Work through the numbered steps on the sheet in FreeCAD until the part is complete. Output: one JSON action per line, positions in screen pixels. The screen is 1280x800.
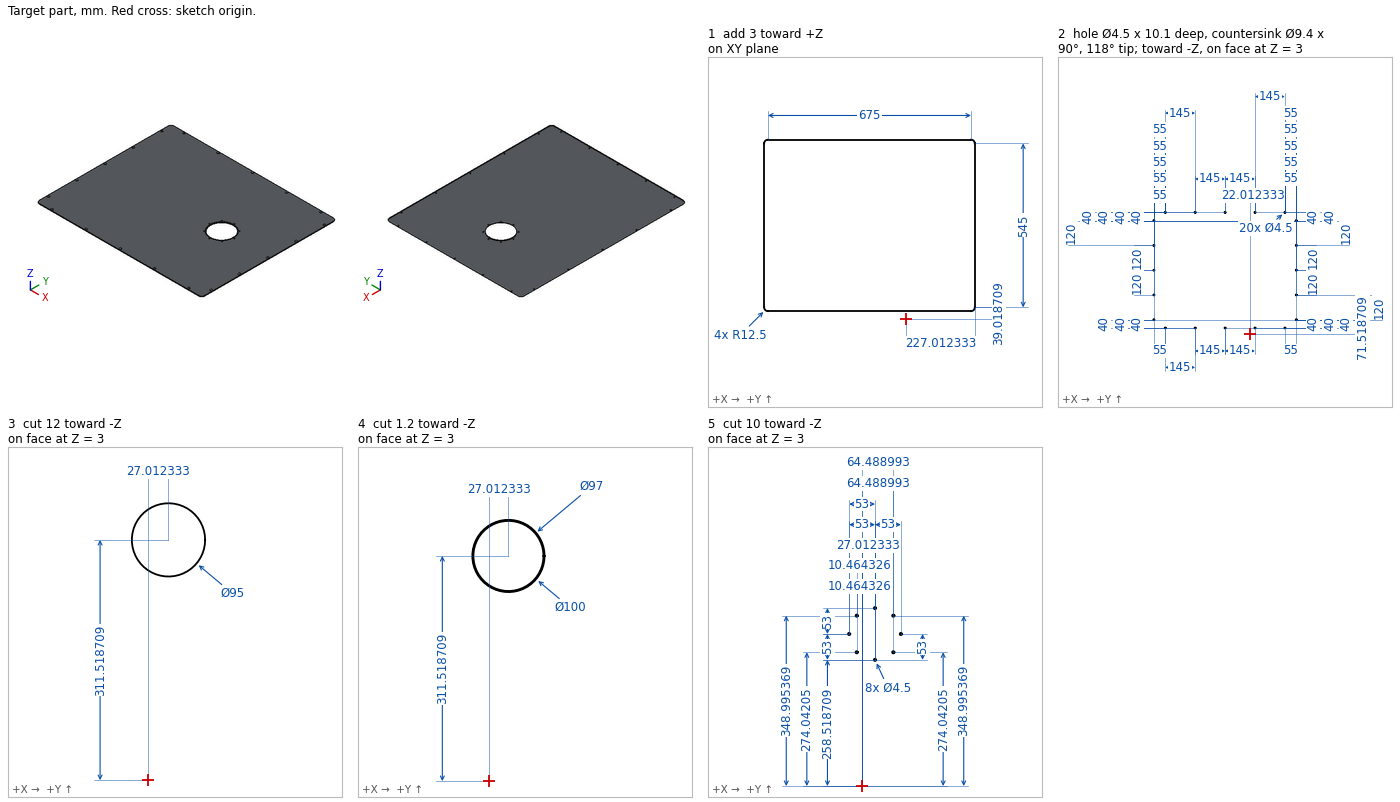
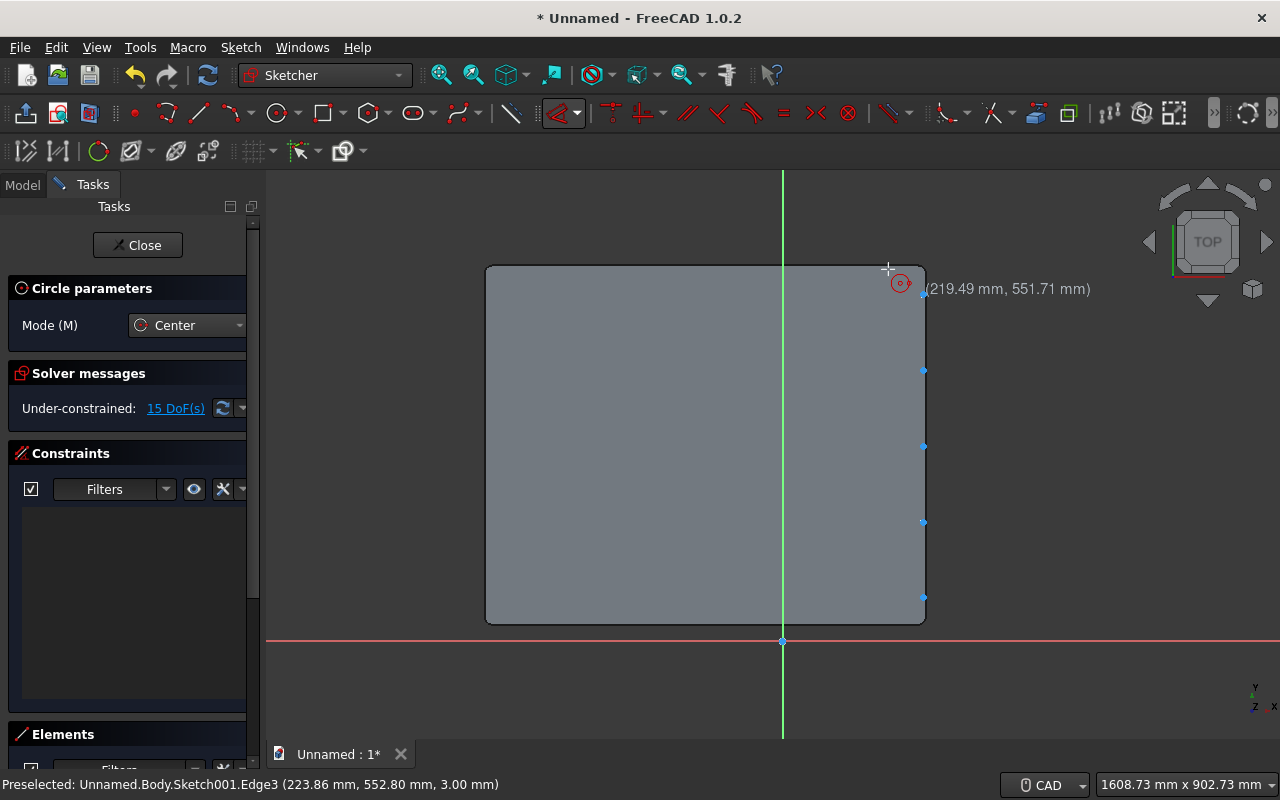
{"action": "left_click", "coordinate": [888, 269]}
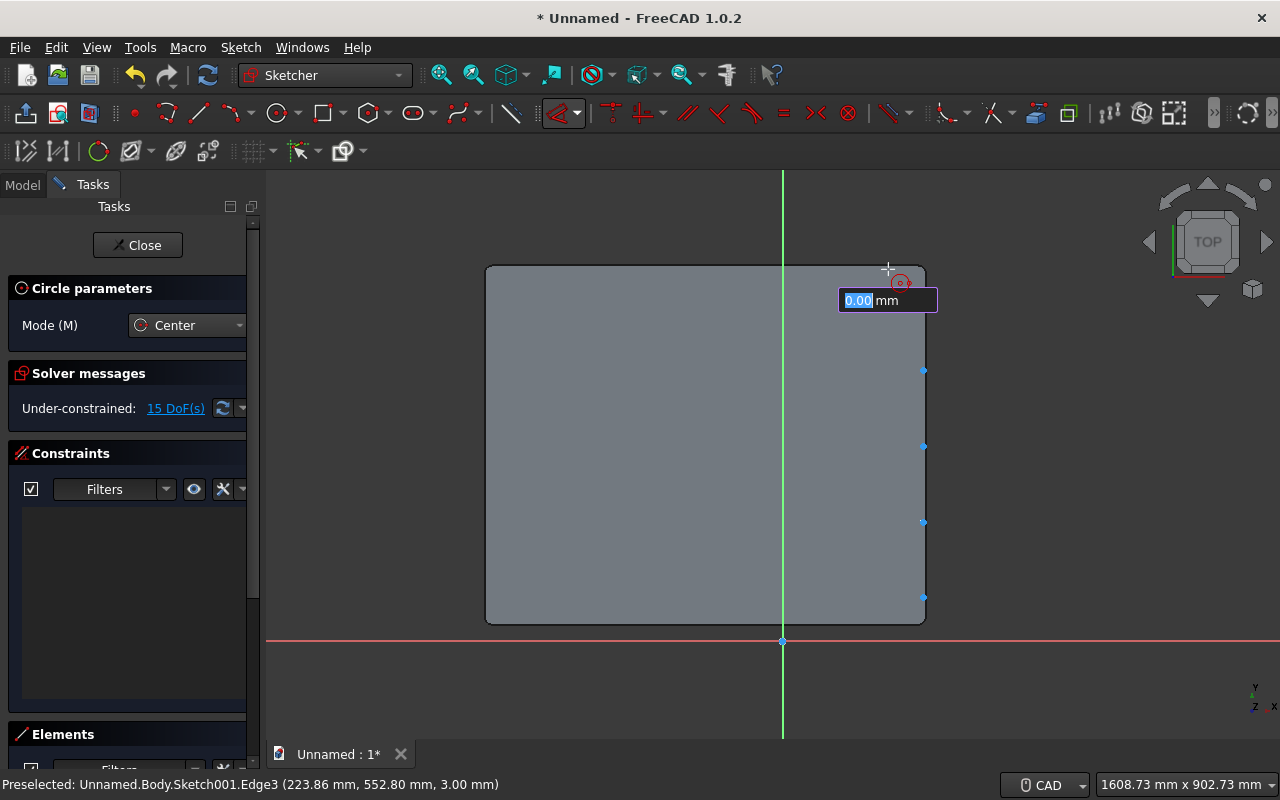
{"action": "scroll", "coordinate": [889, 268], "scroll_direction": "up", "scroll_amount": 13}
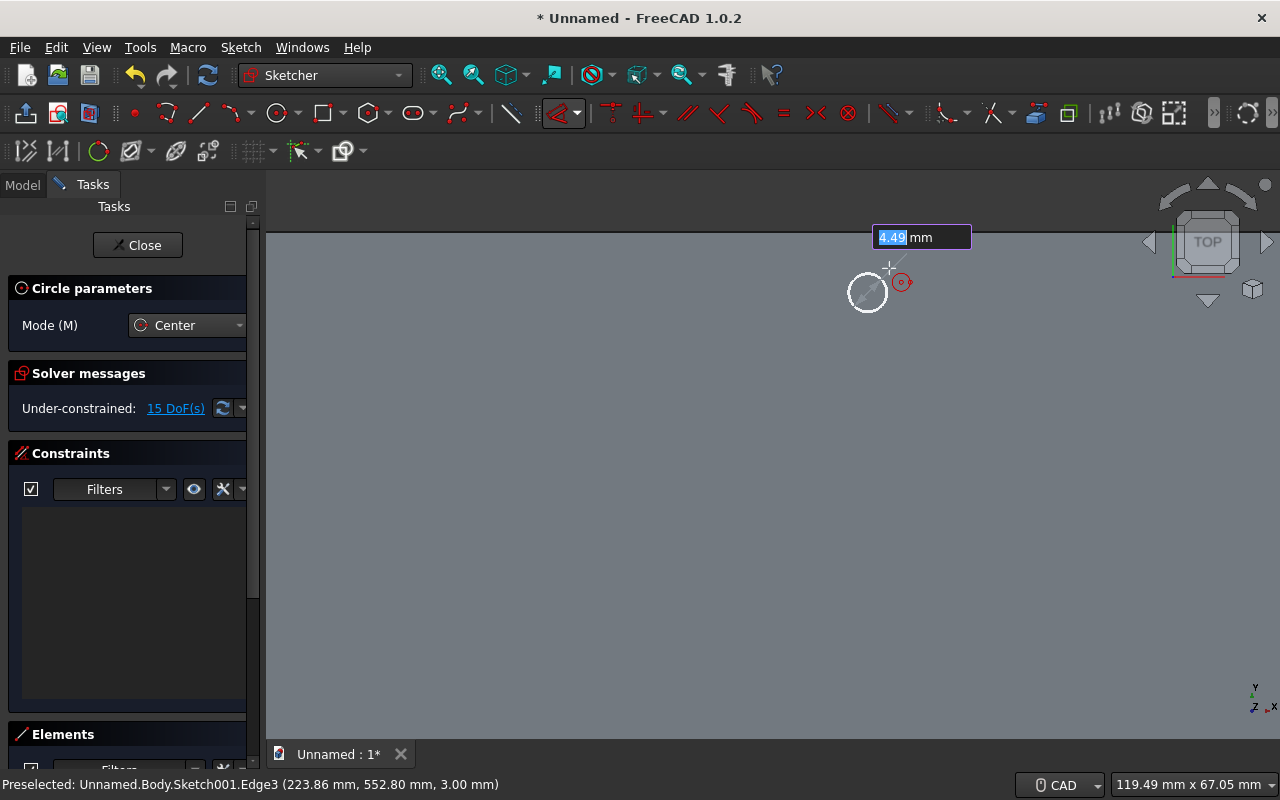
{"action": "left_click", "coordinate": [883, 260]}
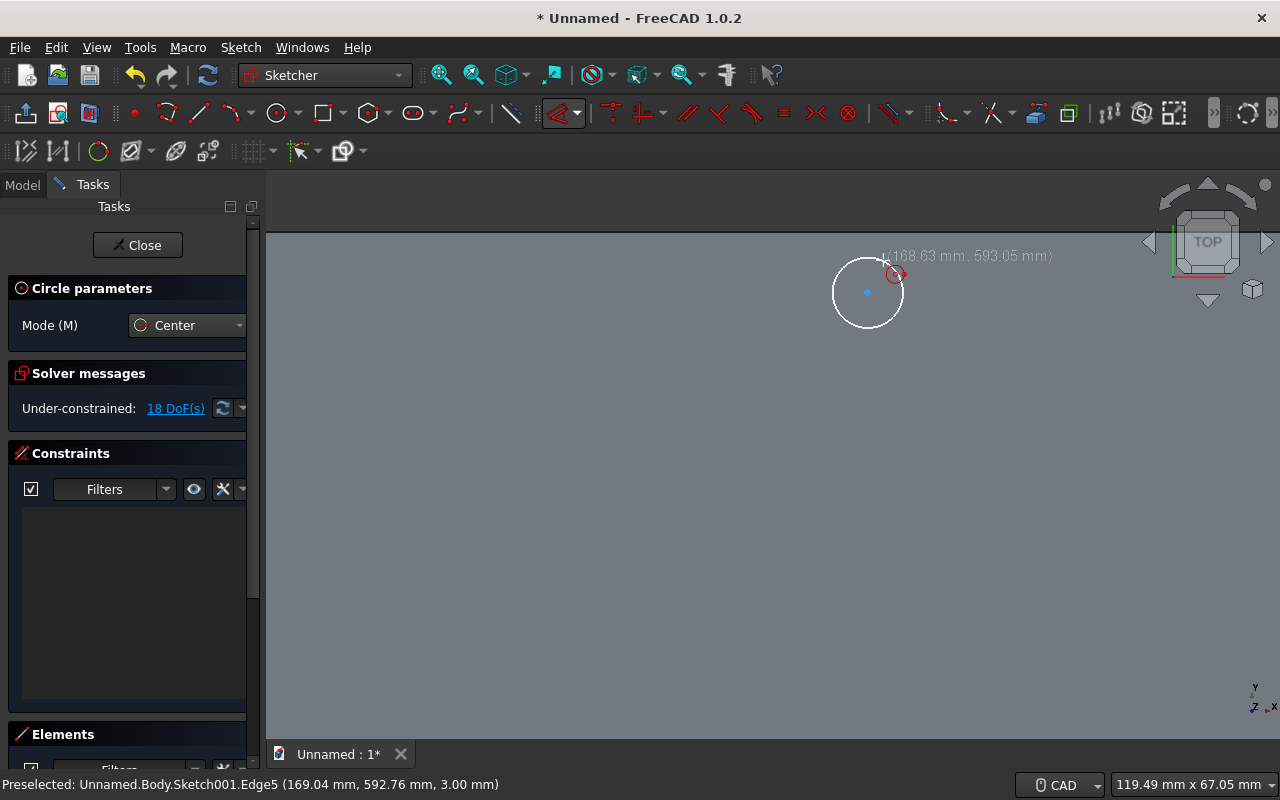
{"action": "scroll", "coordinate": [889, 268], "scroll_direction": "down", "scroll_amount": 13}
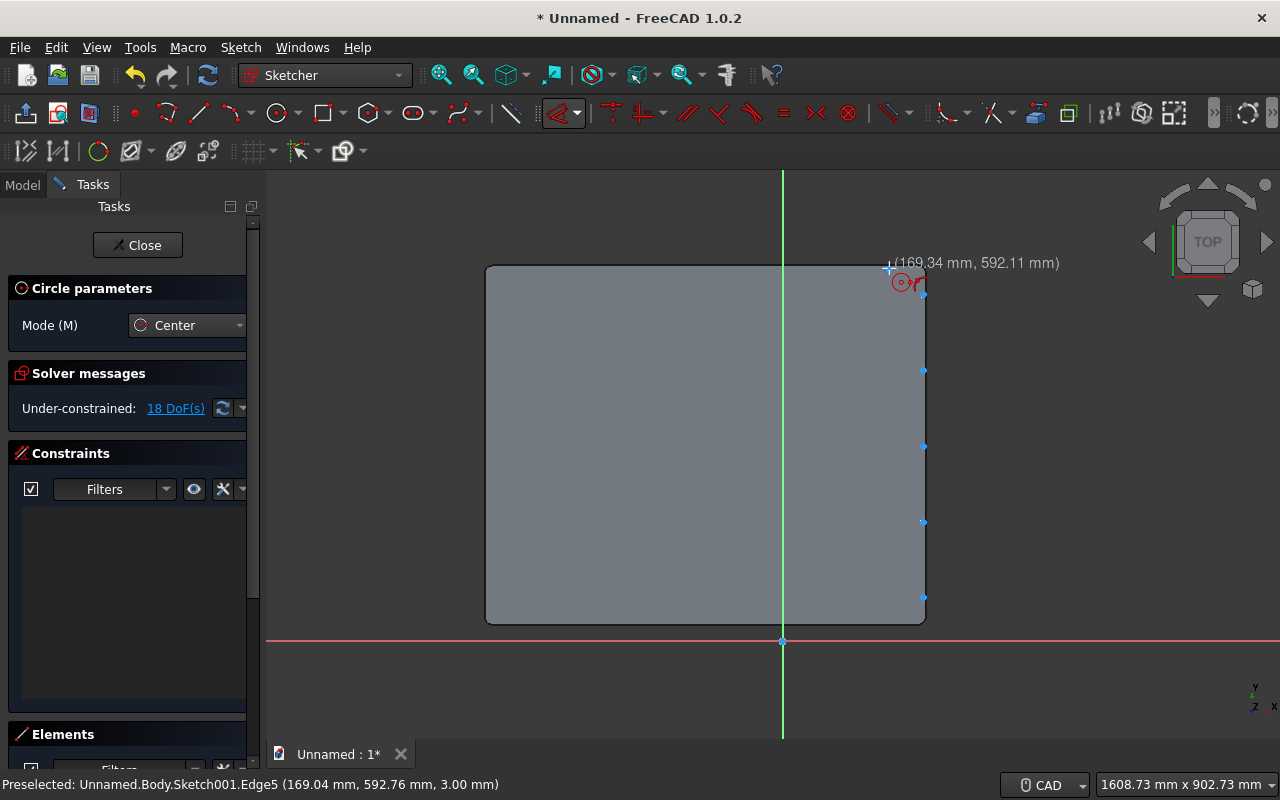
{"action": "scroll", "coordinate": [797, 269], "scroll_direction": "up", "scroll_amount": 14}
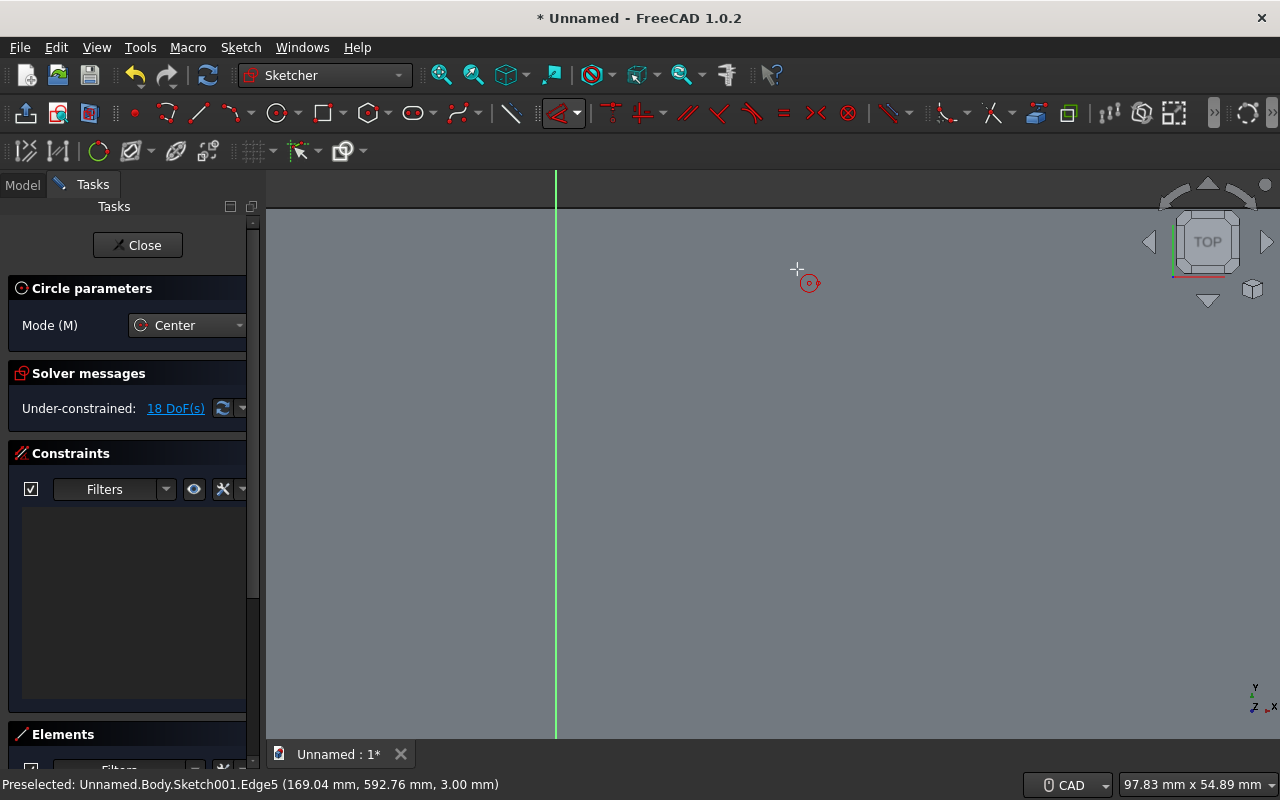
{"action": "scroll", "coordinate": [797, 269], "scroll_direction": "down", "scroll_amount": 14}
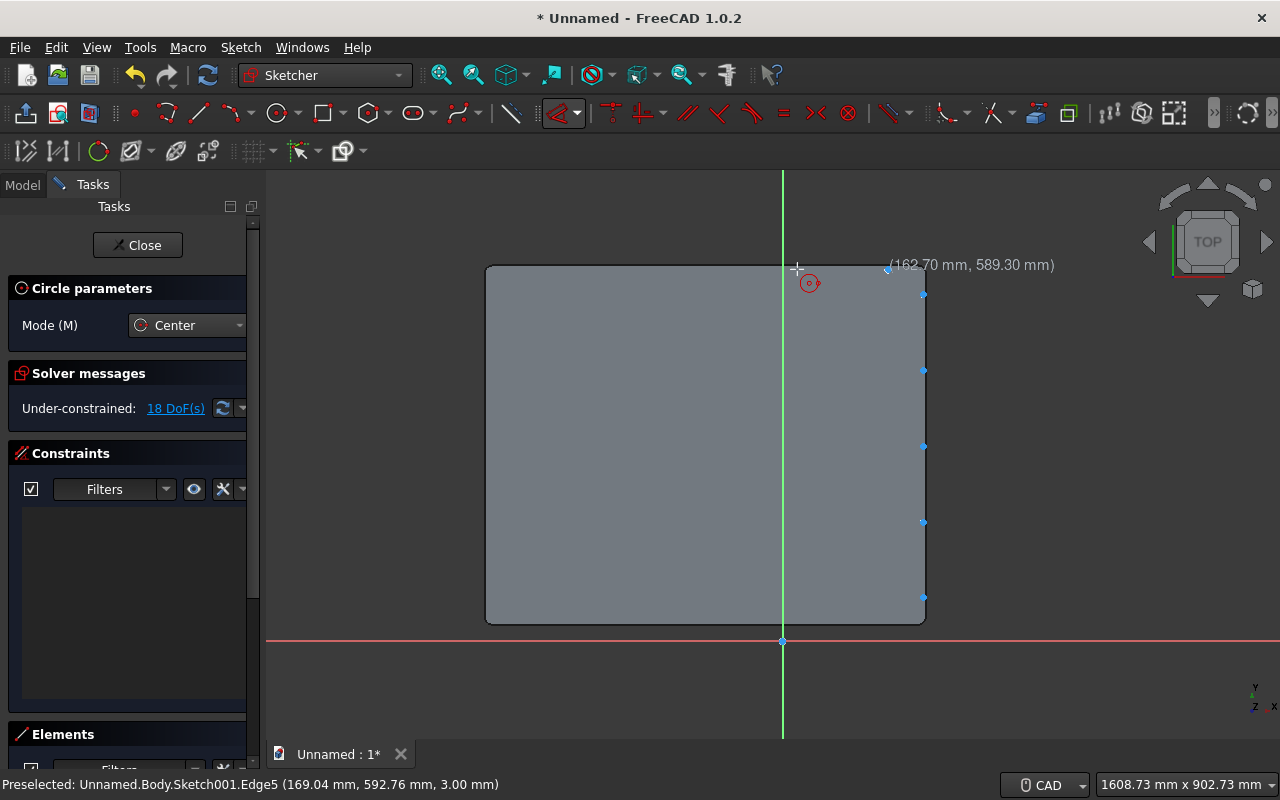
{"action": "left_click", "coordinate": [797, 269]}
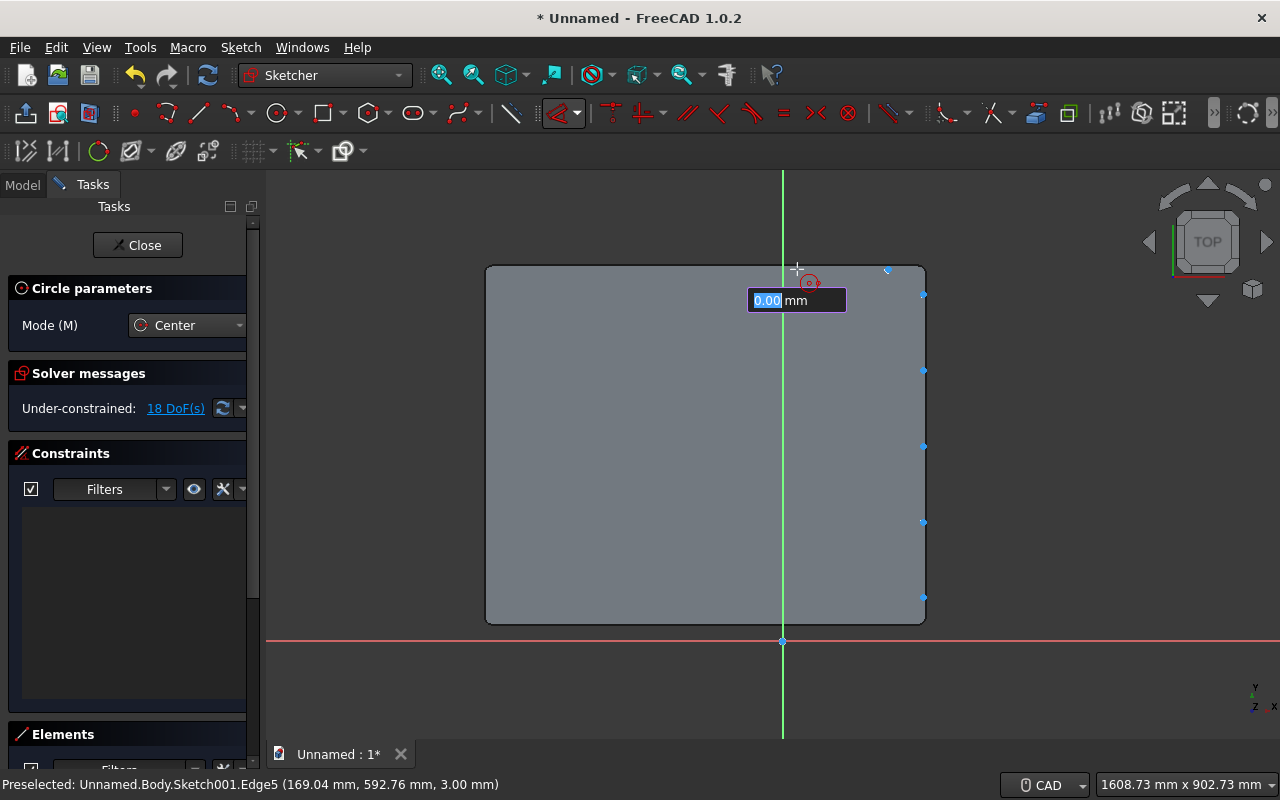
{"action": "scroll", "coordinate": [798, 268], "scroll_direction": "up", "scroll_amount": 13}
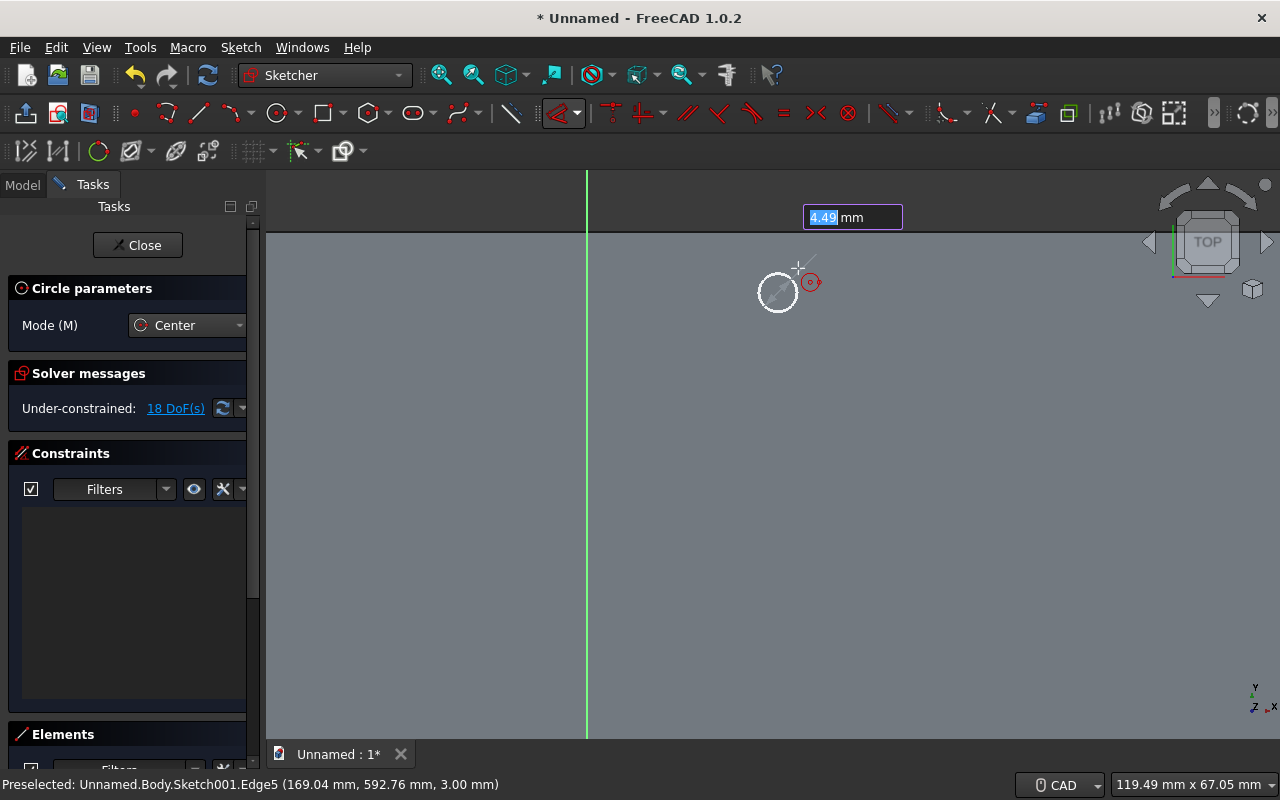
{"action": "left_click", "coordinate": [788, 260]}